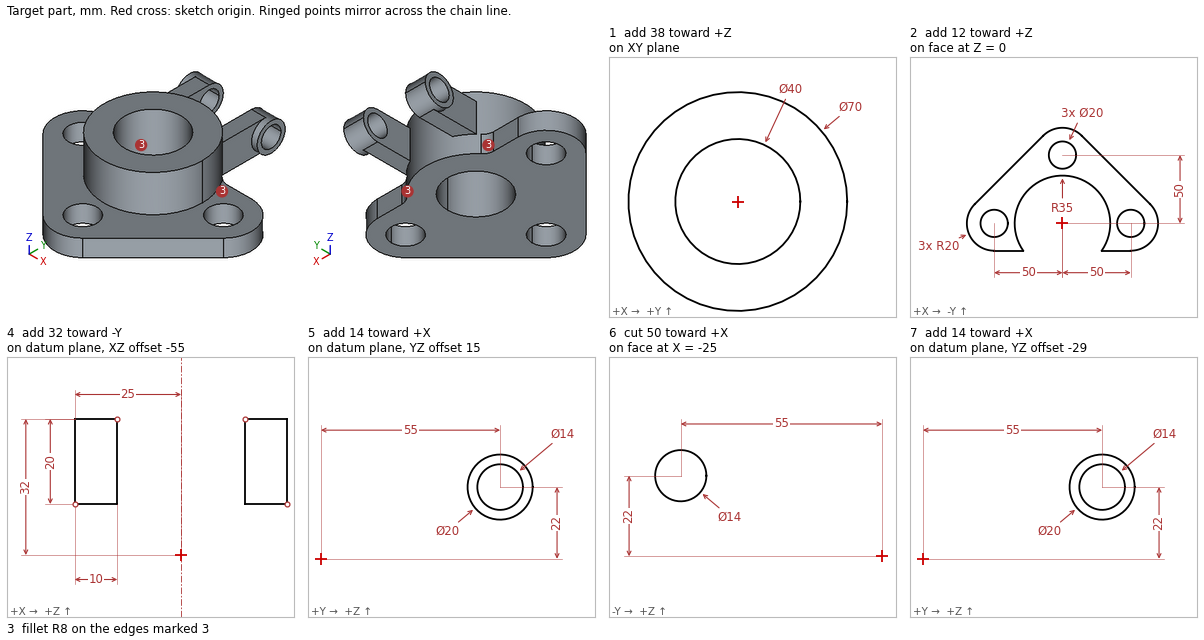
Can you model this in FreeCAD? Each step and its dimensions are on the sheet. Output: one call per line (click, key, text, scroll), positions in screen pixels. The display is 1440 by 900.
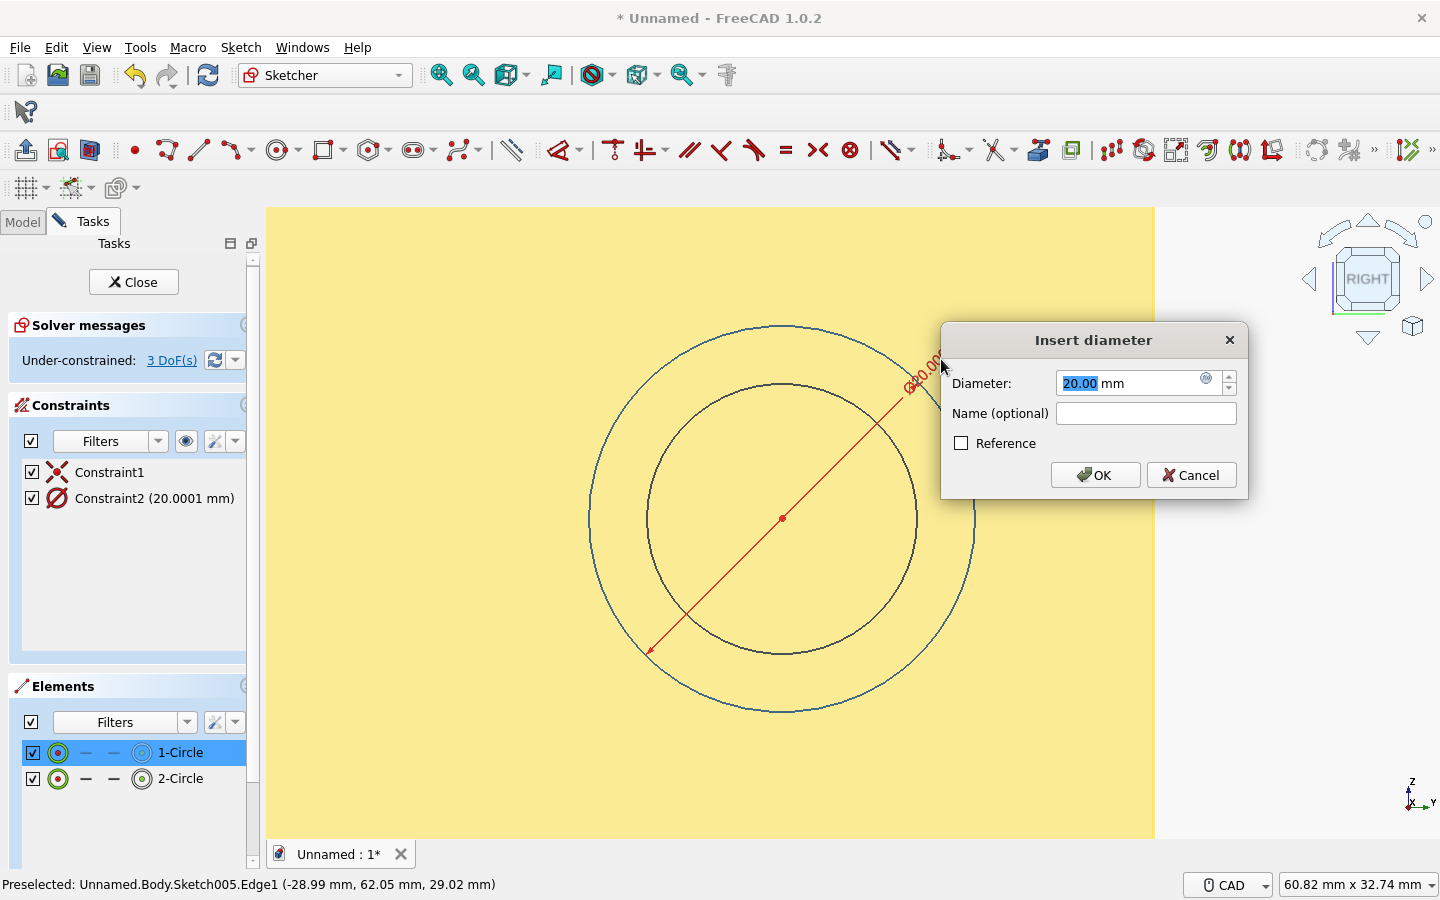
text(20)
key(Return)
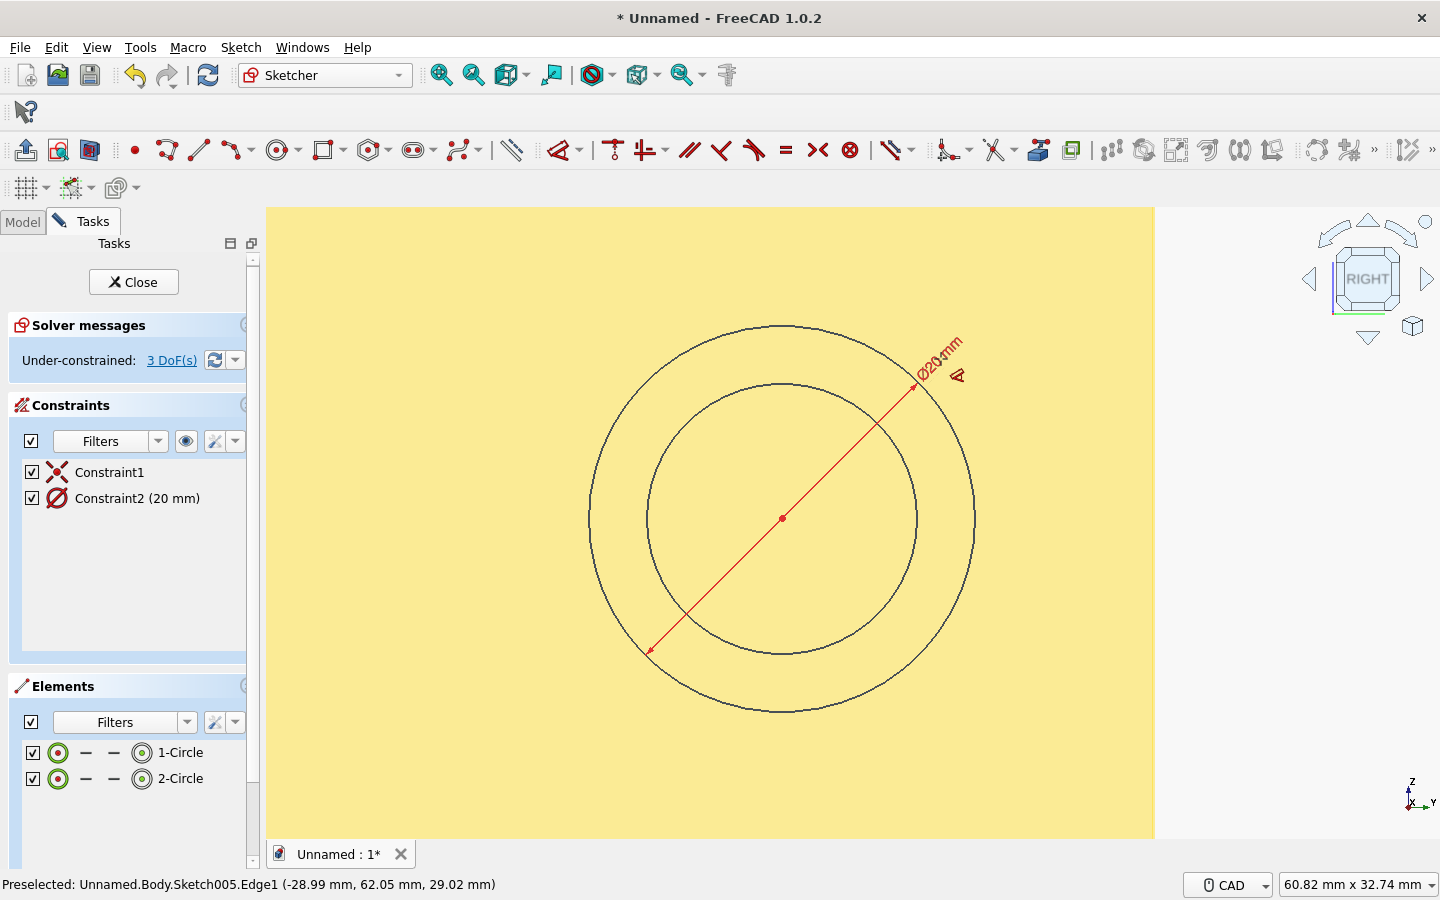
click(877, 423)
click(900, 400)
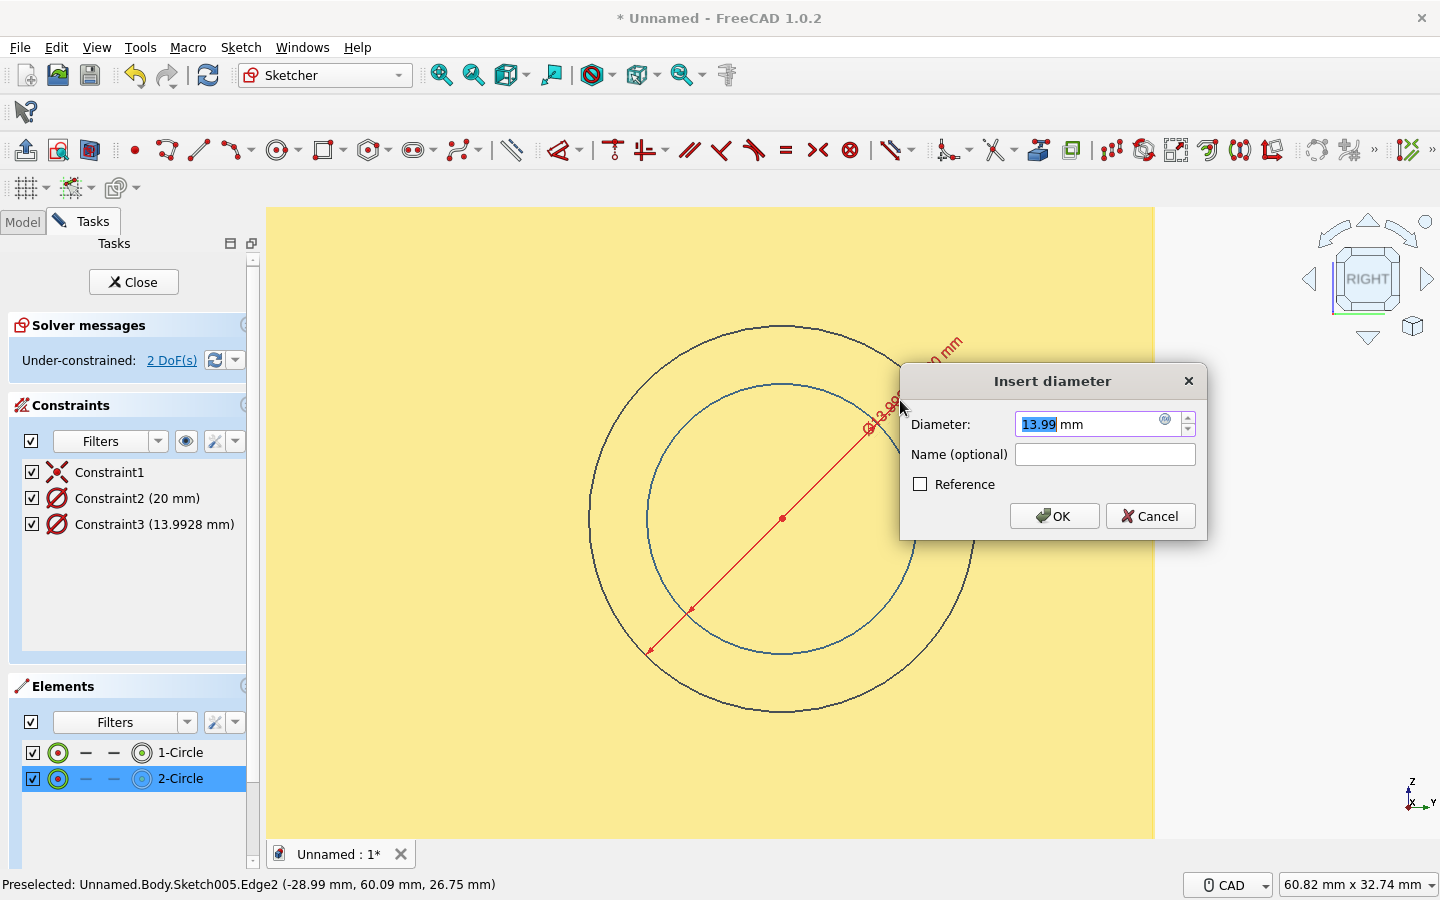
text(14)
key(Return)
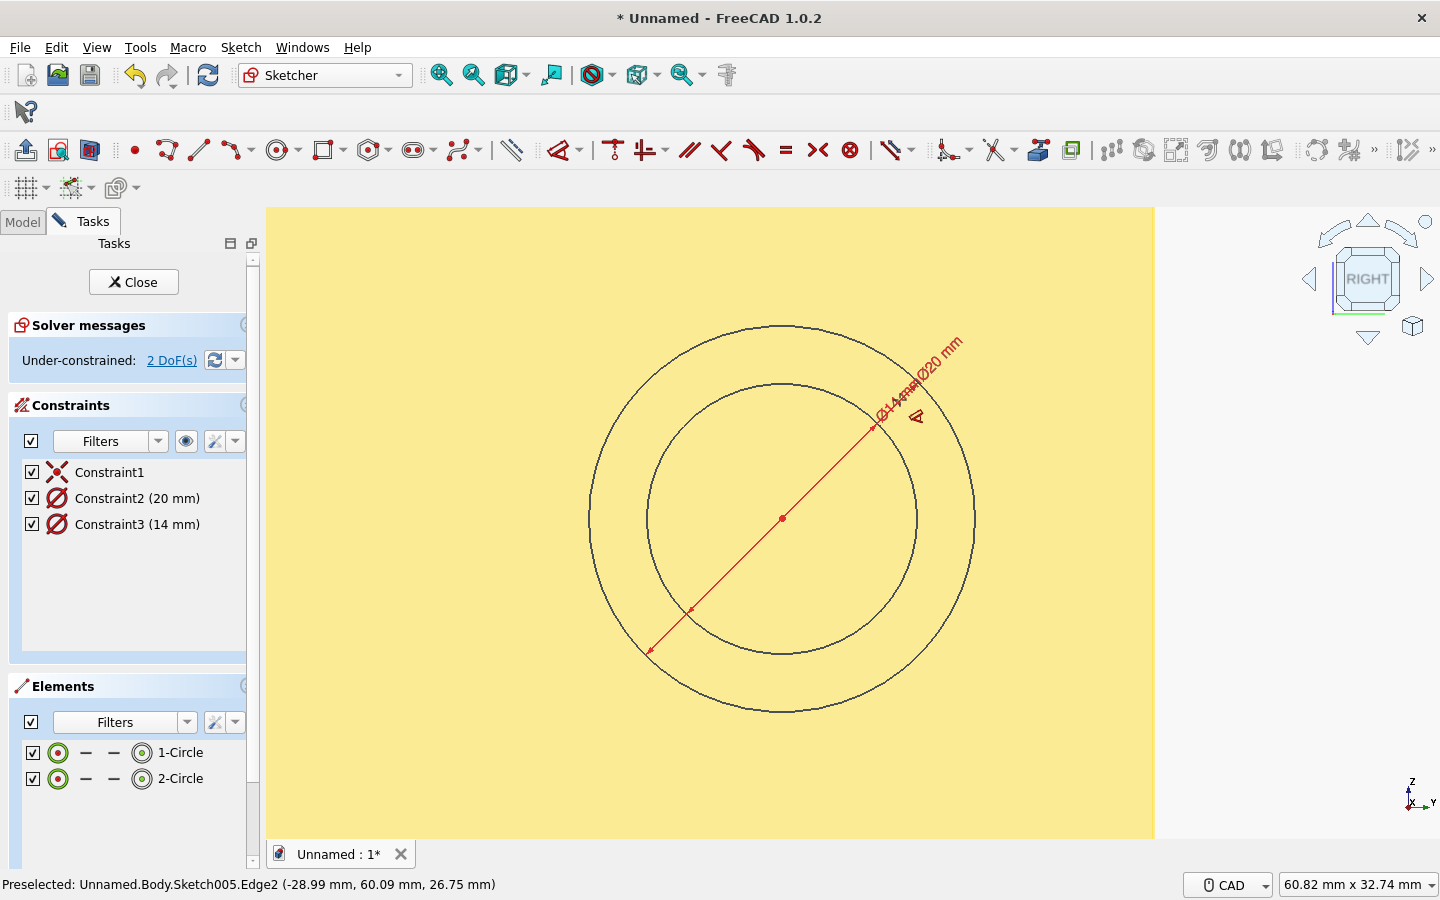
click(782, 519)
click(538, 485)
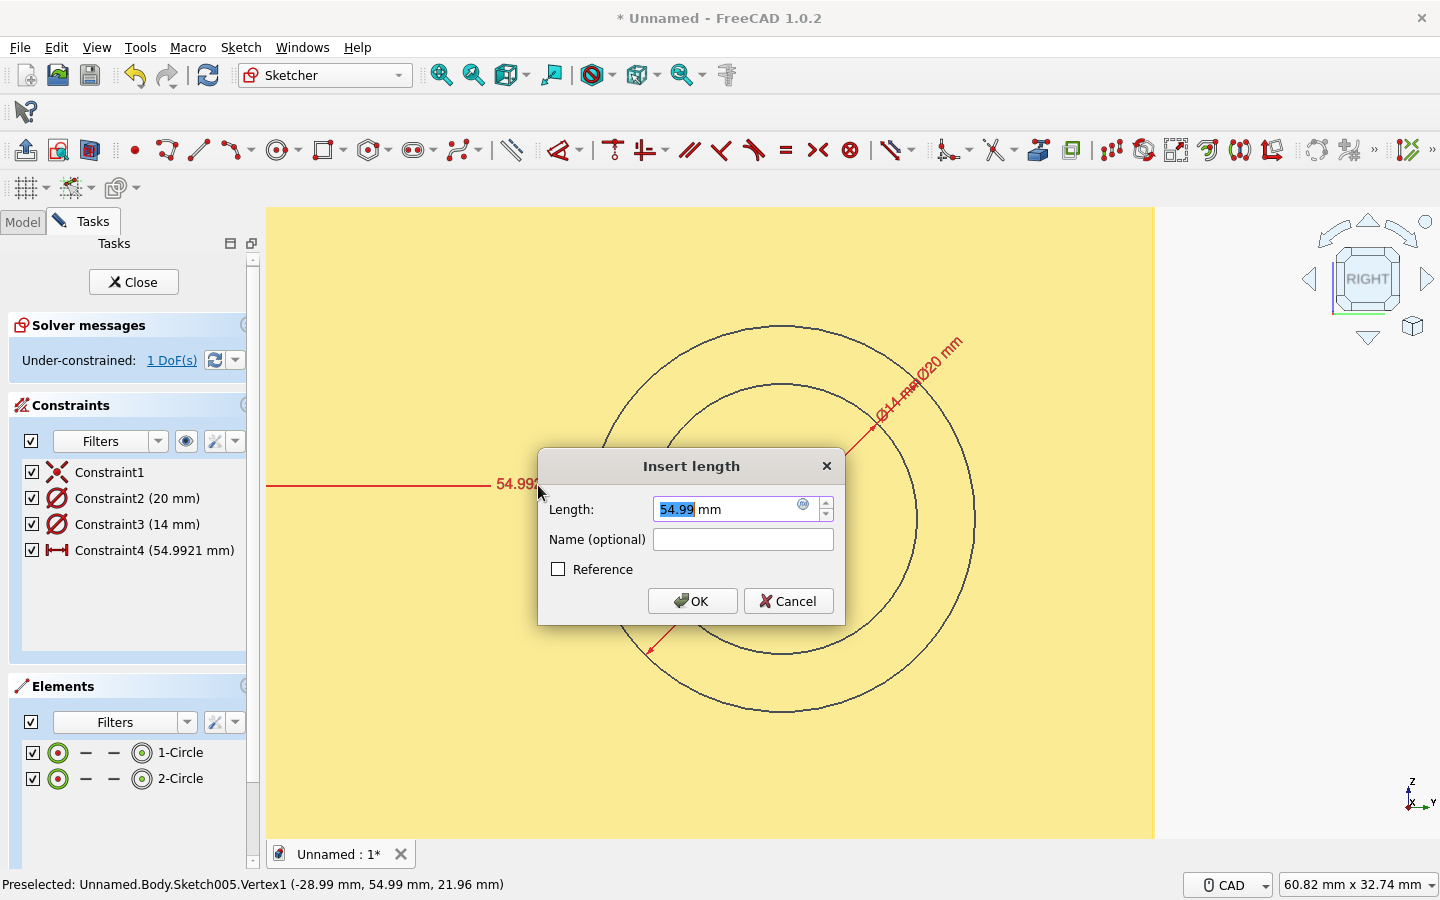
text(55)
key(Return)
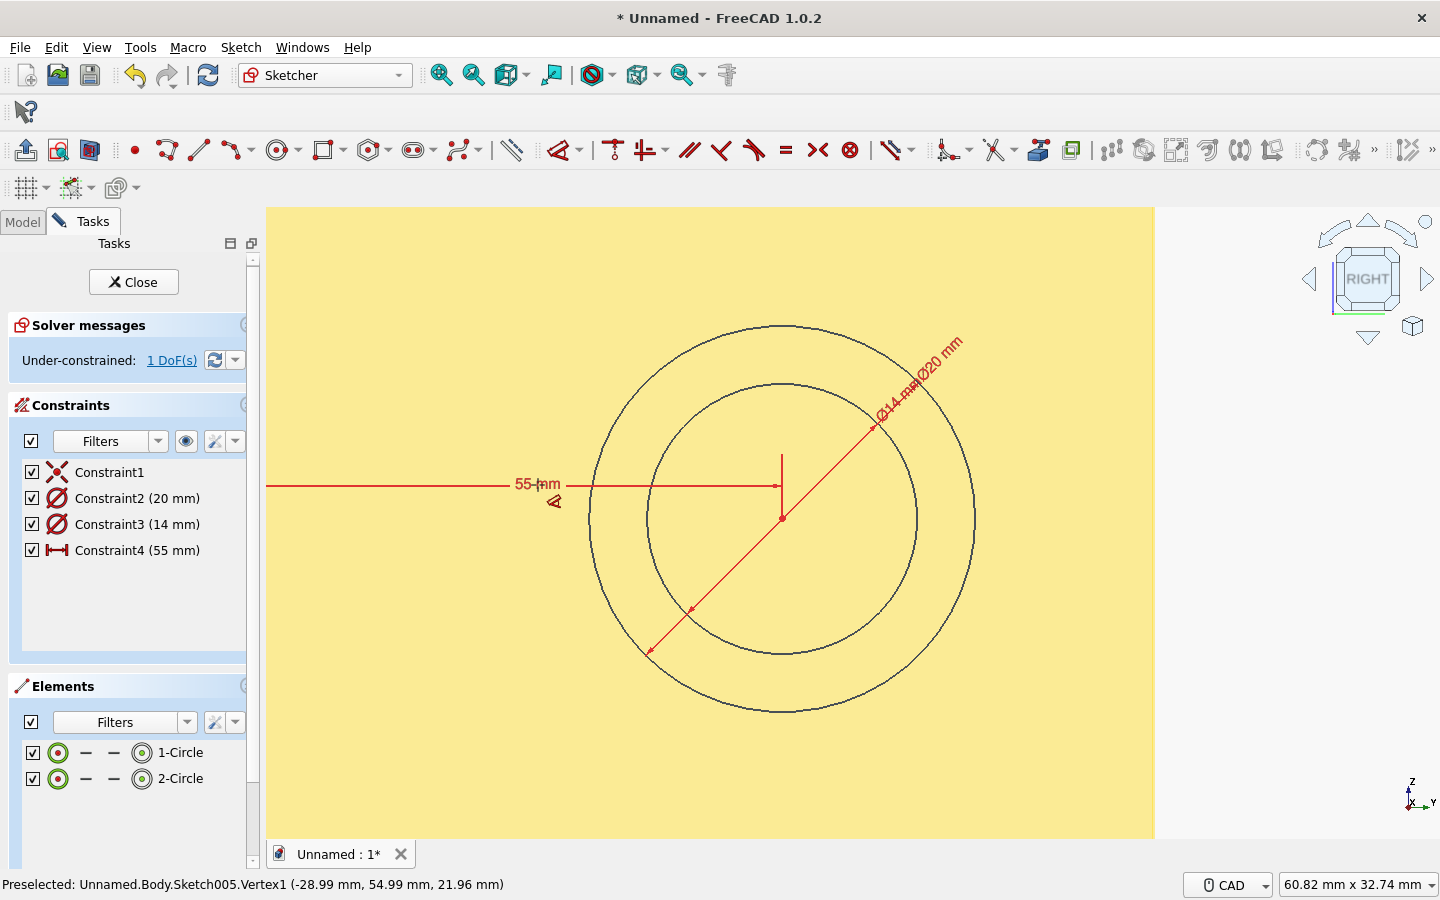
click(782, 519)
click(816, 665)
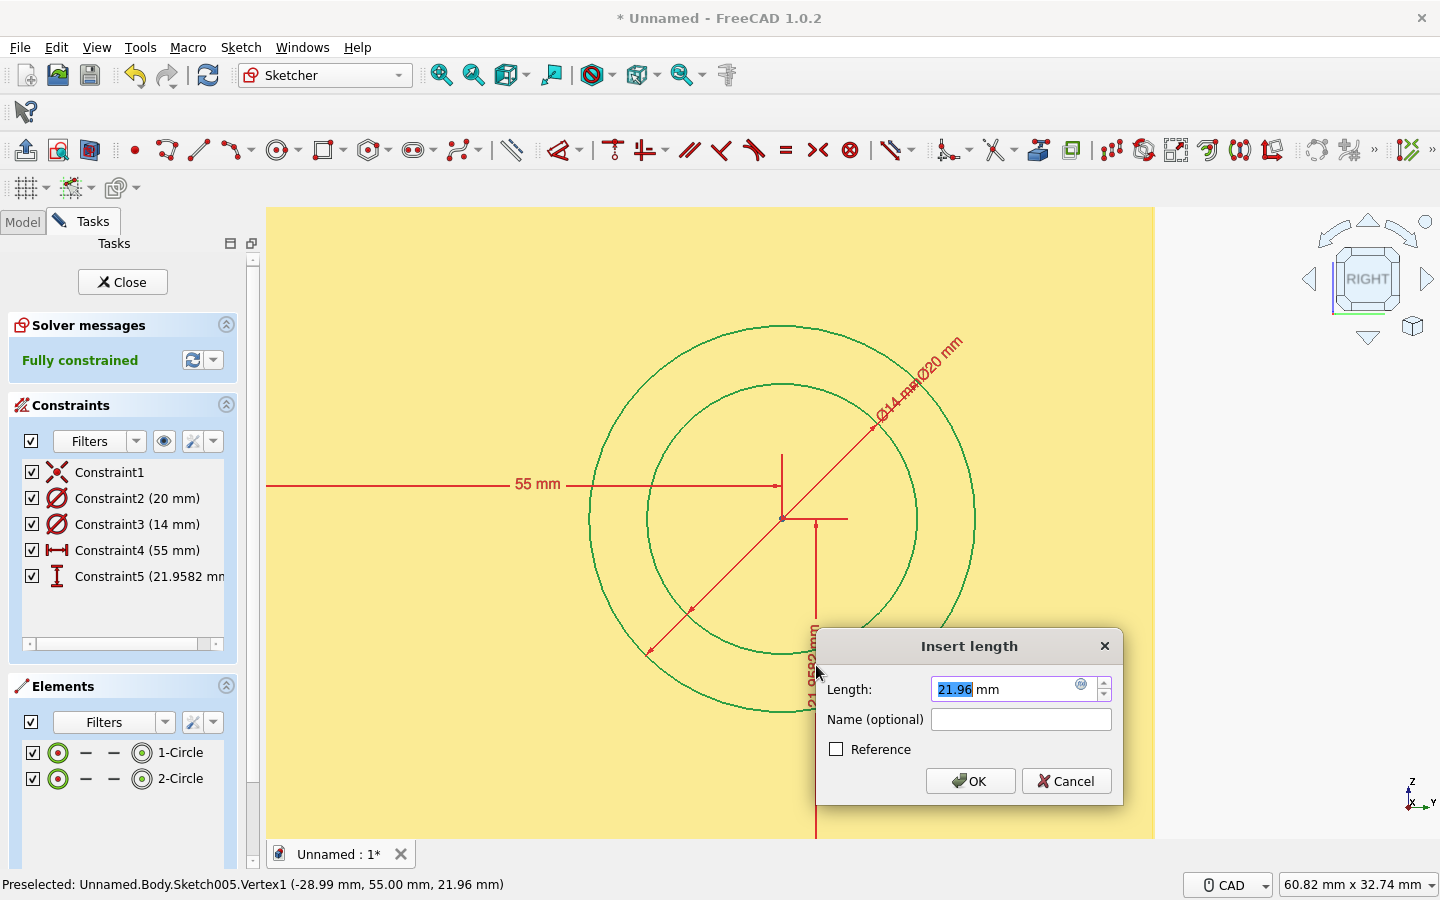
text(22)
key(Return)
key(Escape)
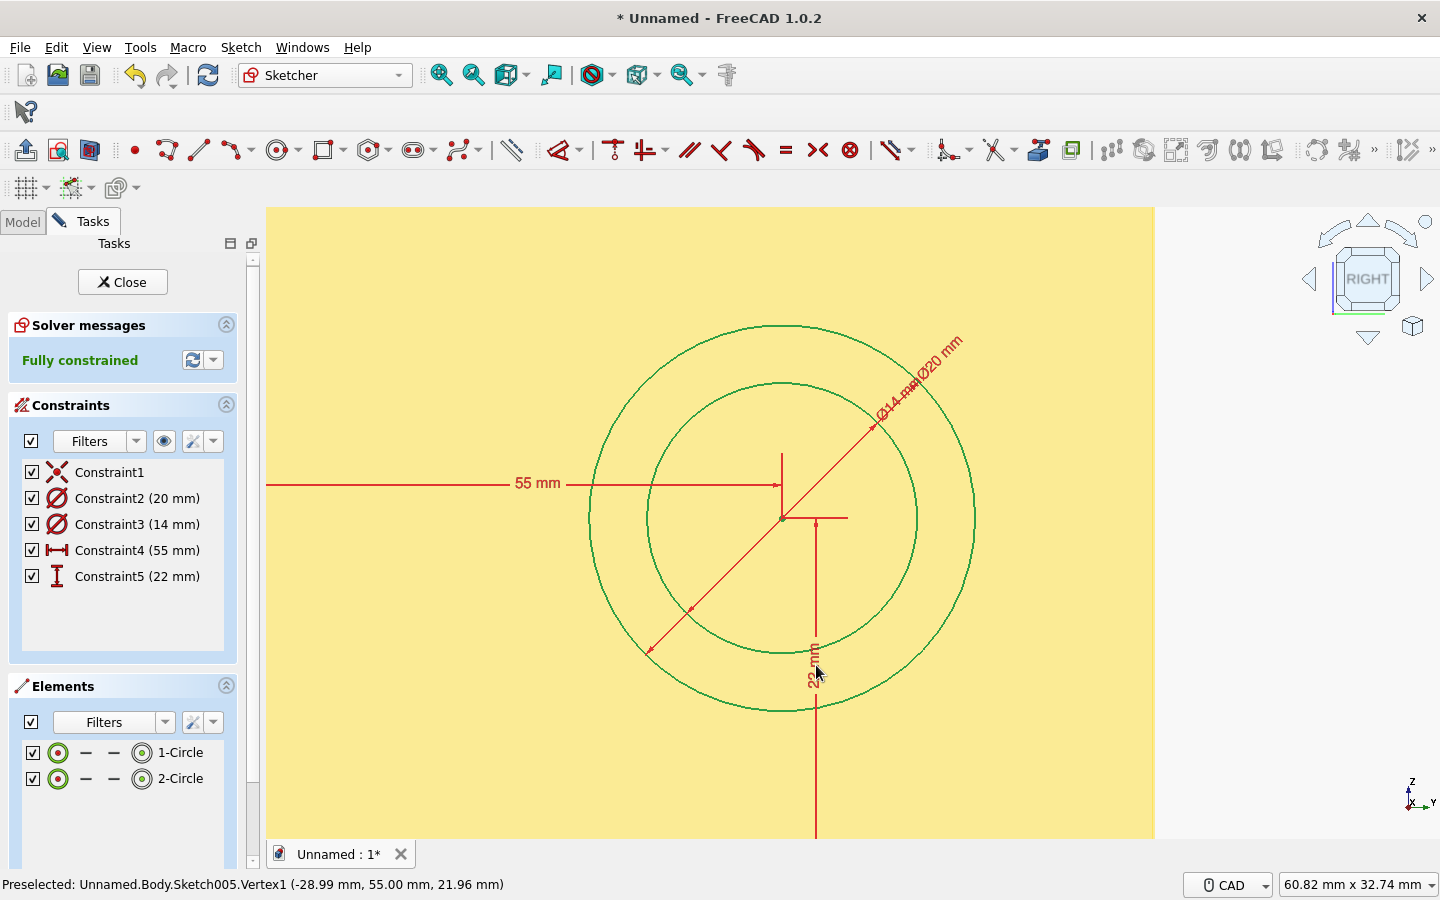
click(123, 282)